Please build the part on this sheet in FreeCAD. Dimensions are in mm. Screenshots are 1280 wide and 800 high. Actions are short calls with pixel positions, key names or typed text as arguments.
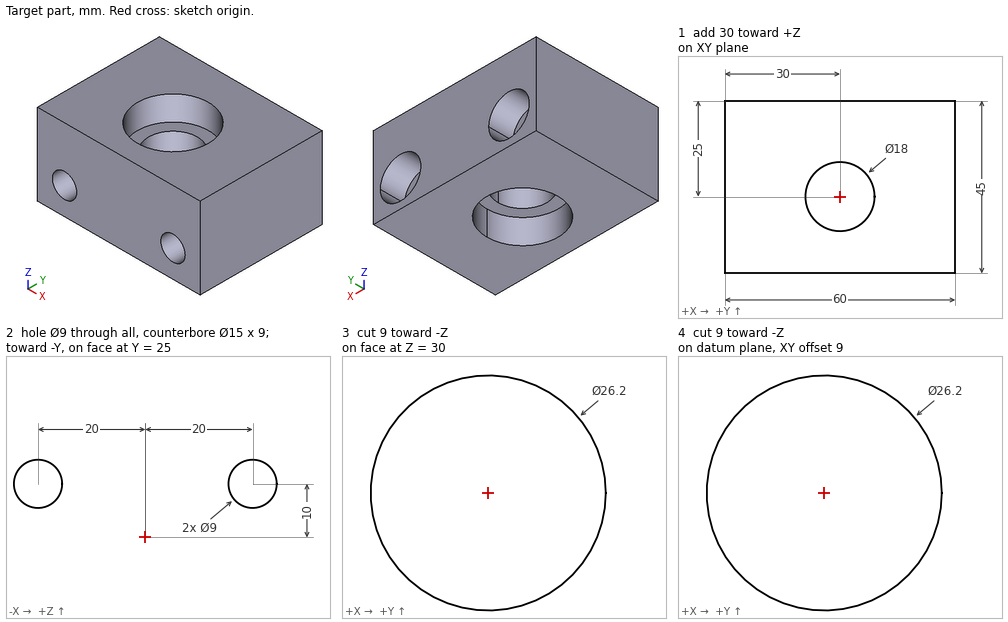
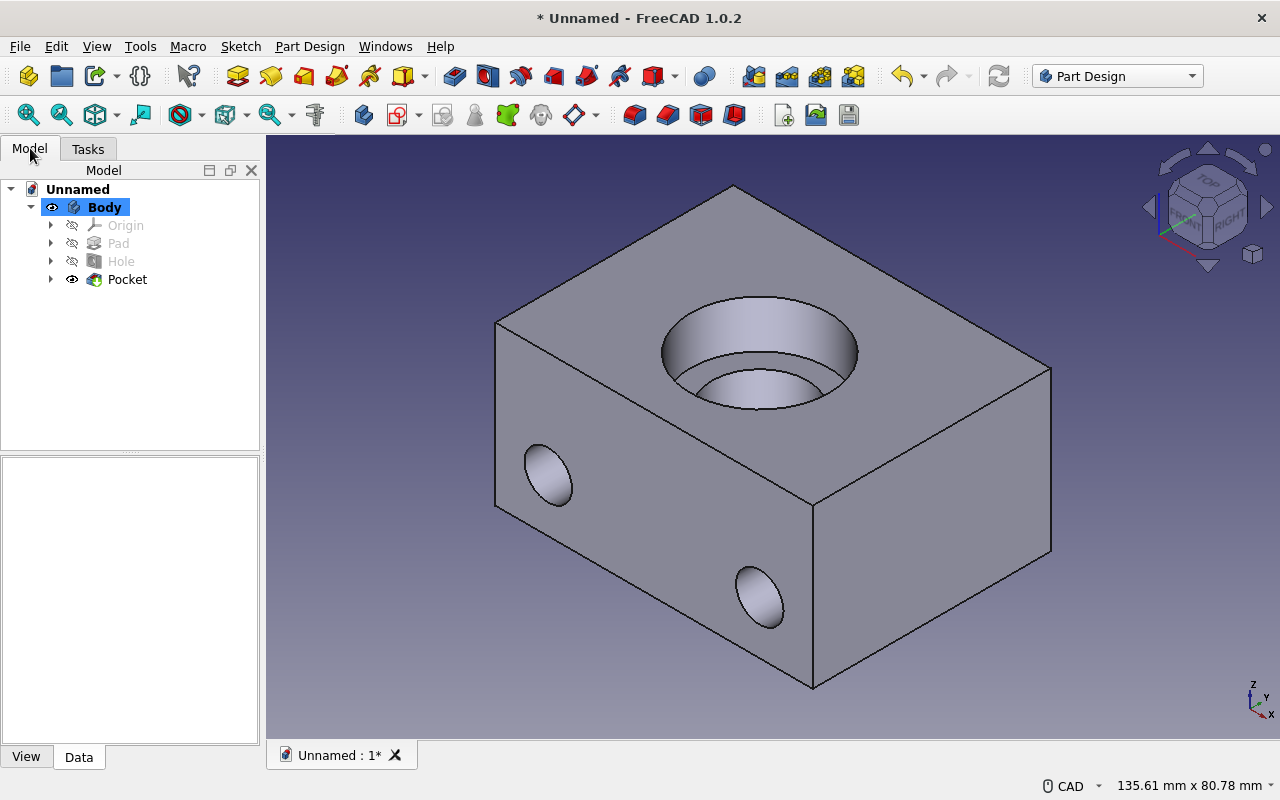
click(51, 225)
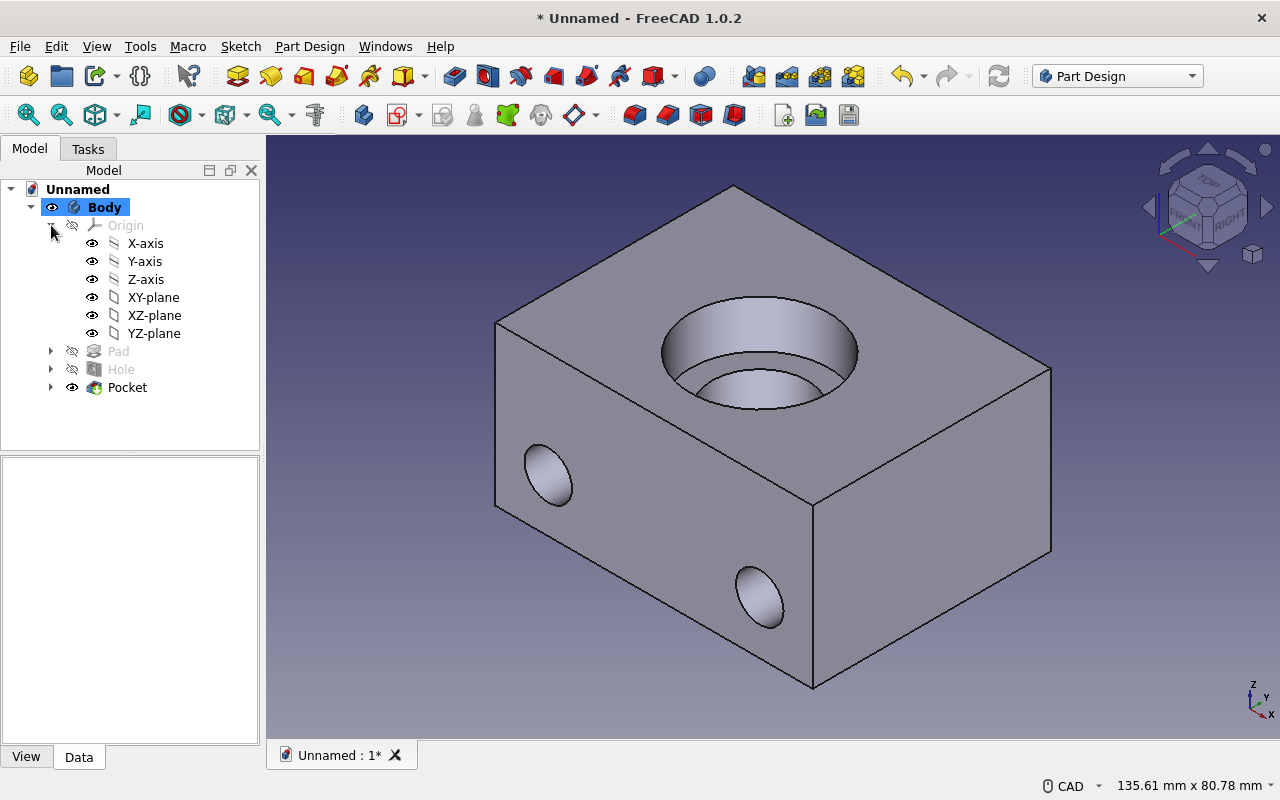
click(137, 297)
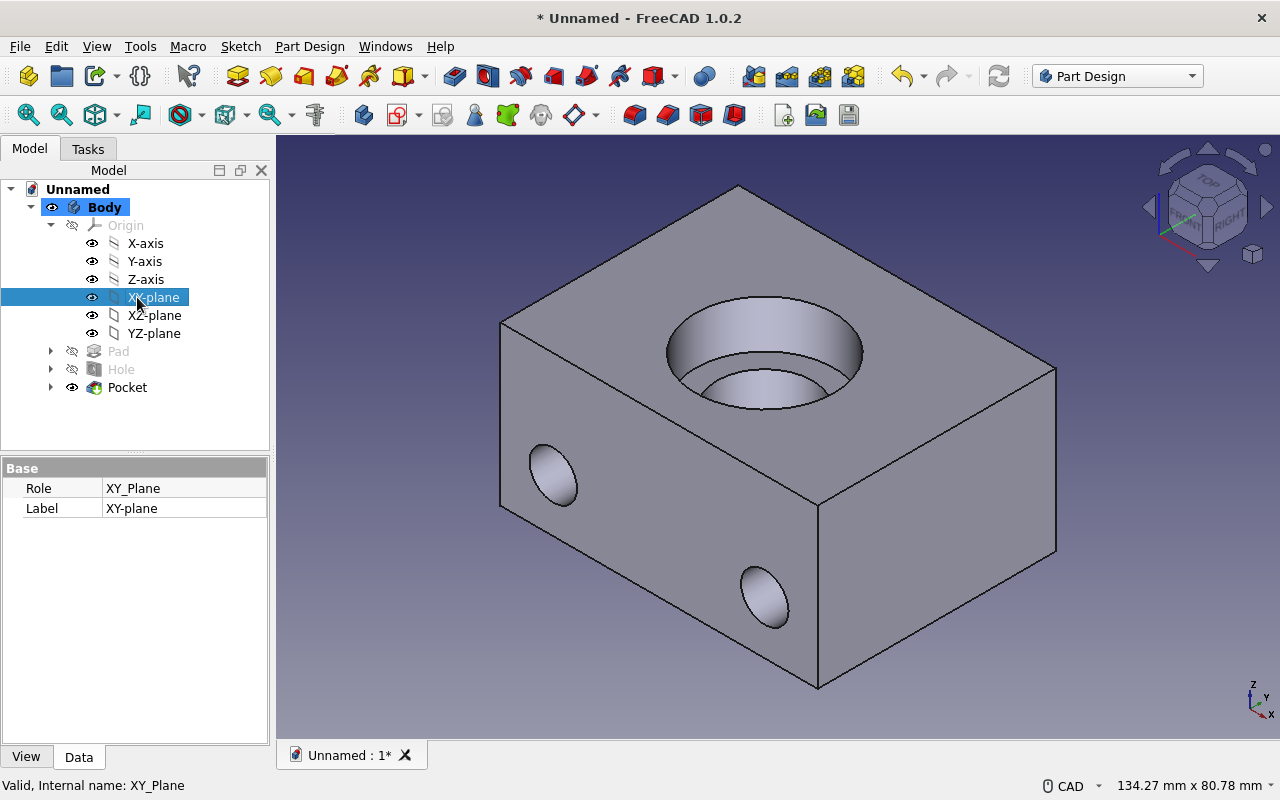
click(574, 116)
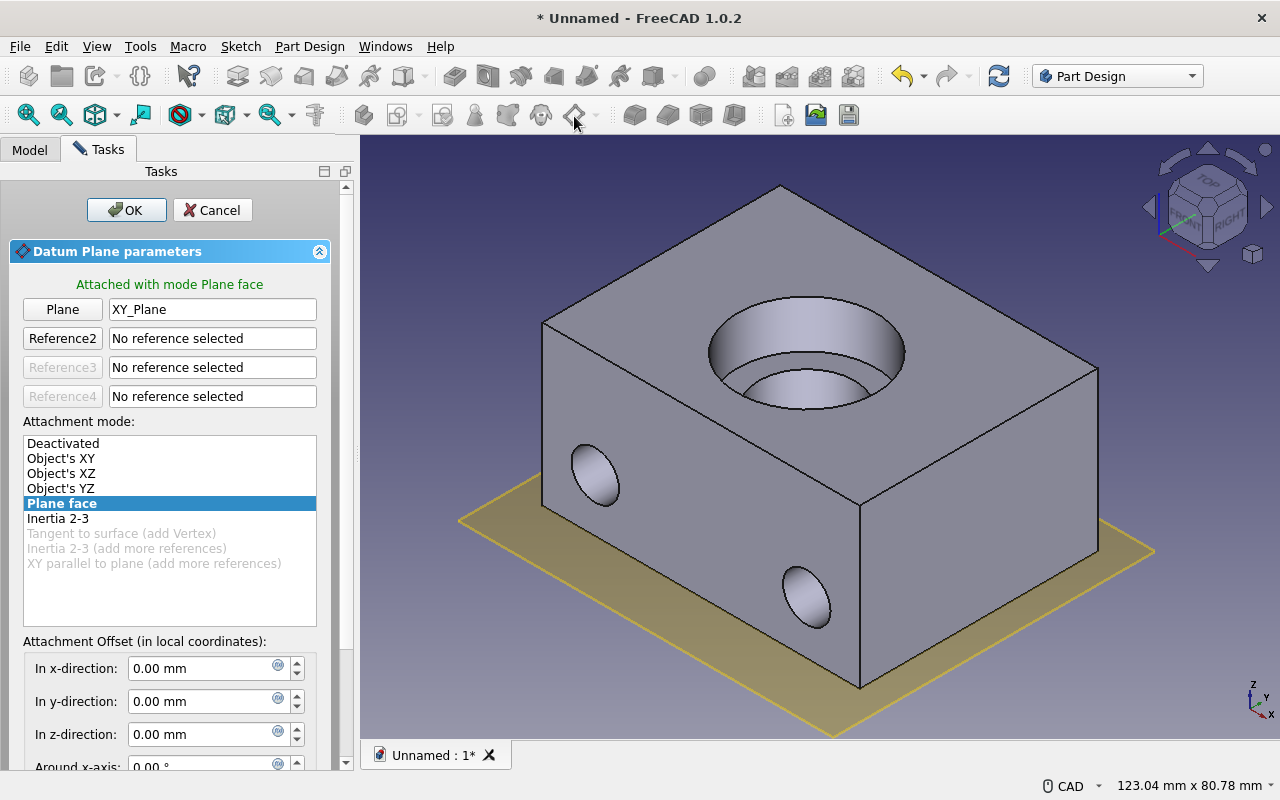
triple_click(210, 734)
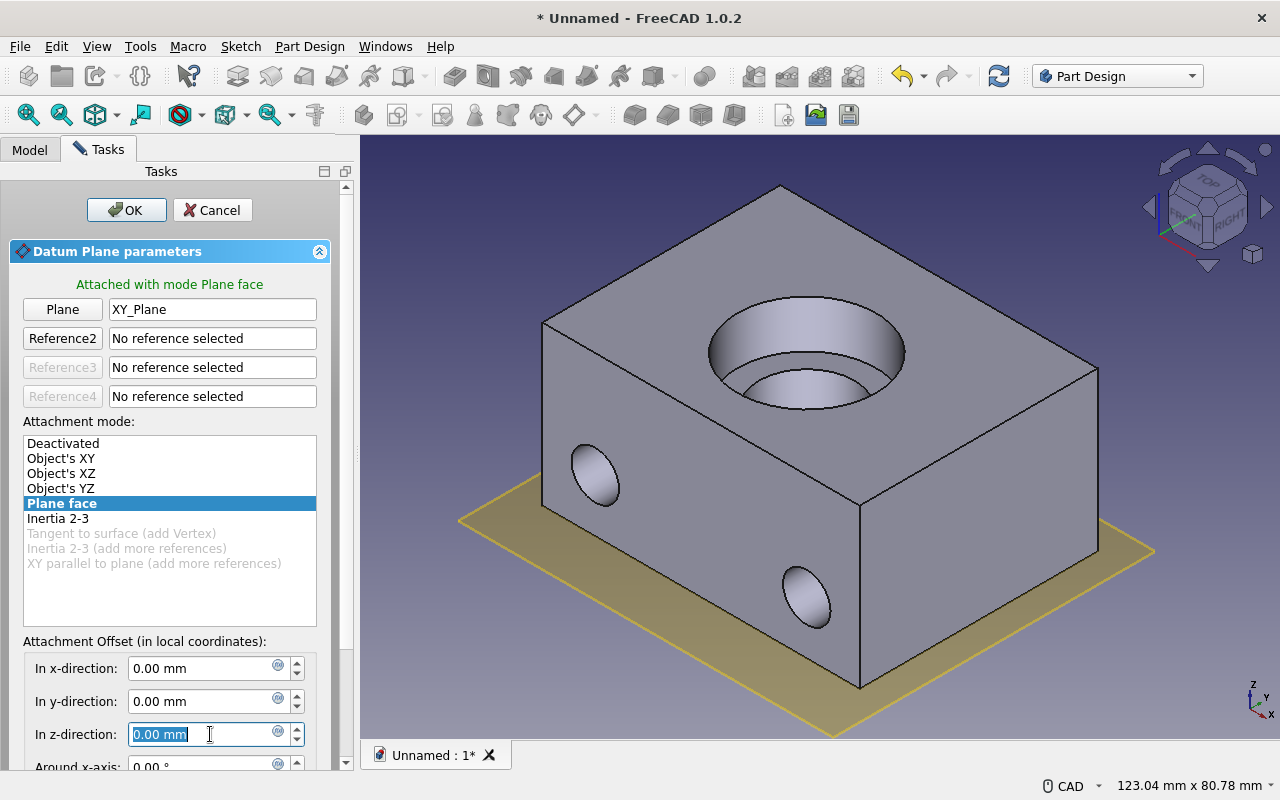
text(9)
key(Tab)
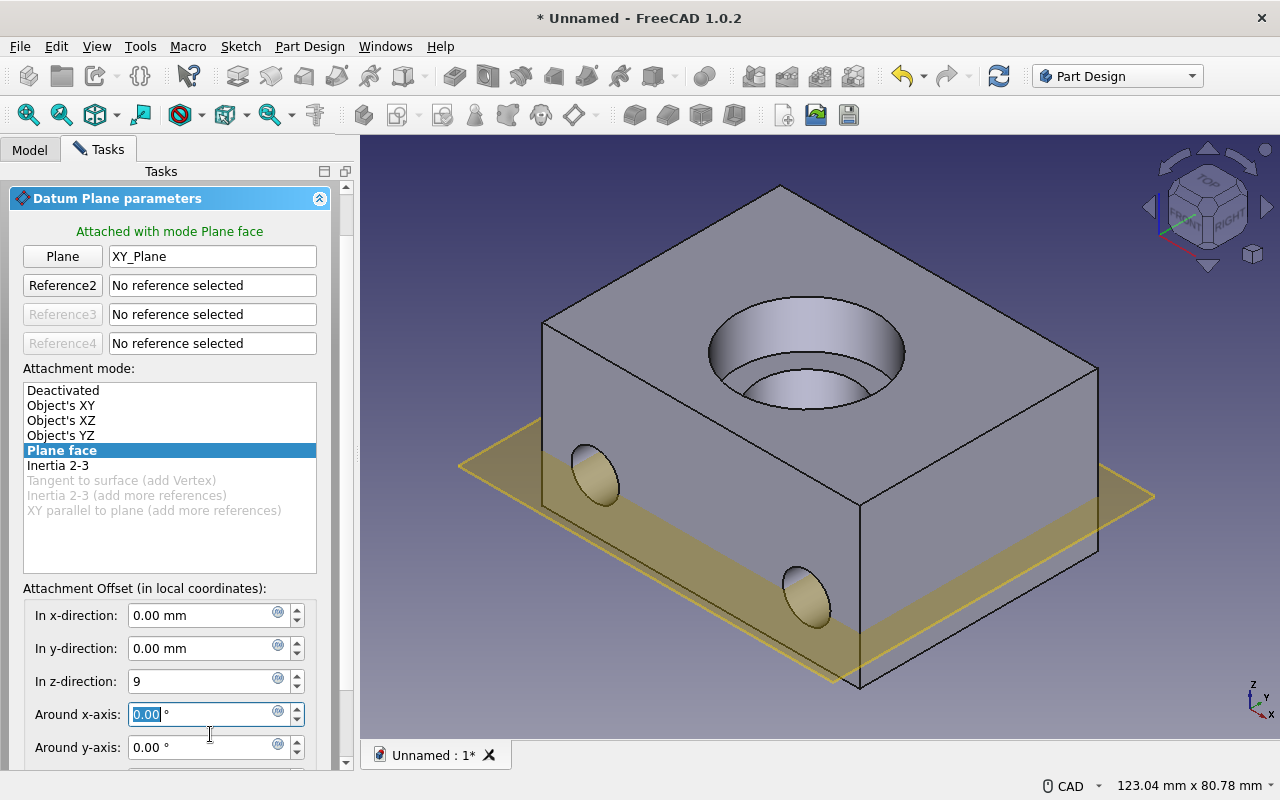
scroll(346, 476, up, 2)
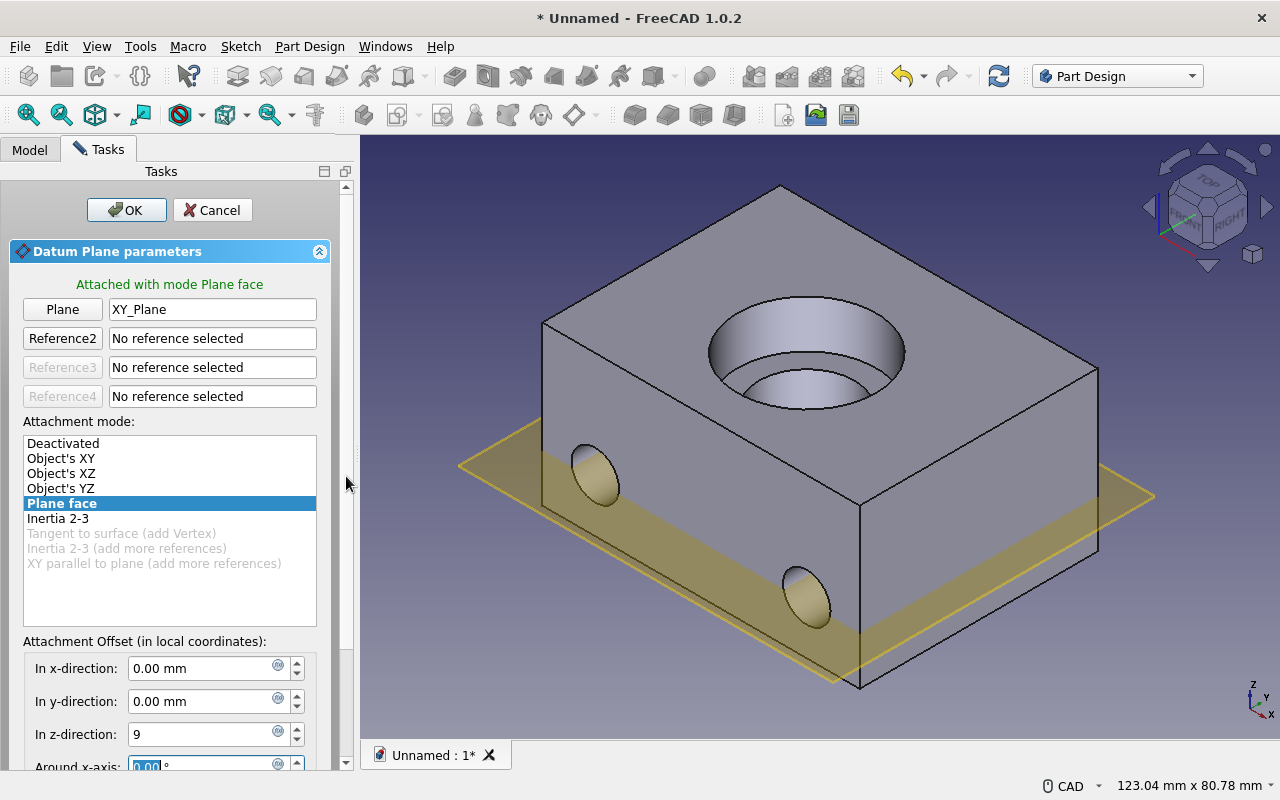
click(127, 210)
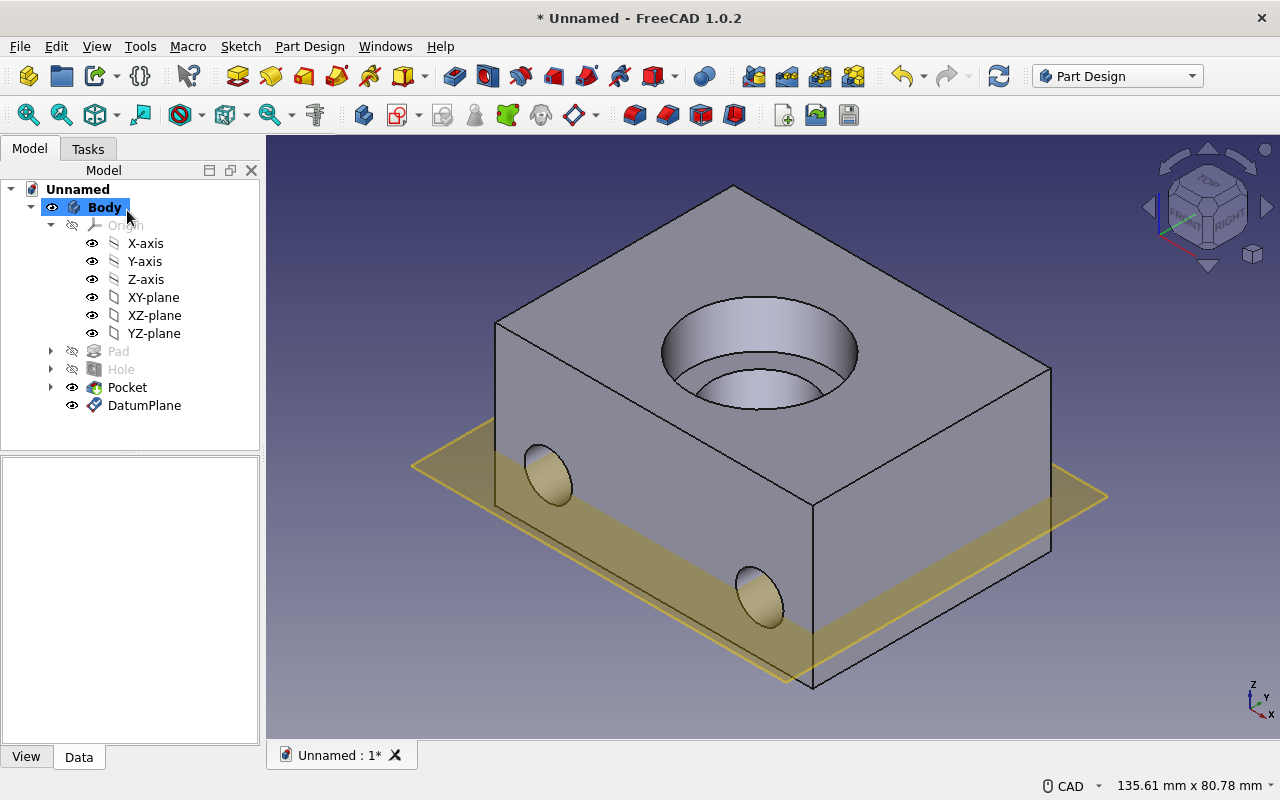
click(117, 405)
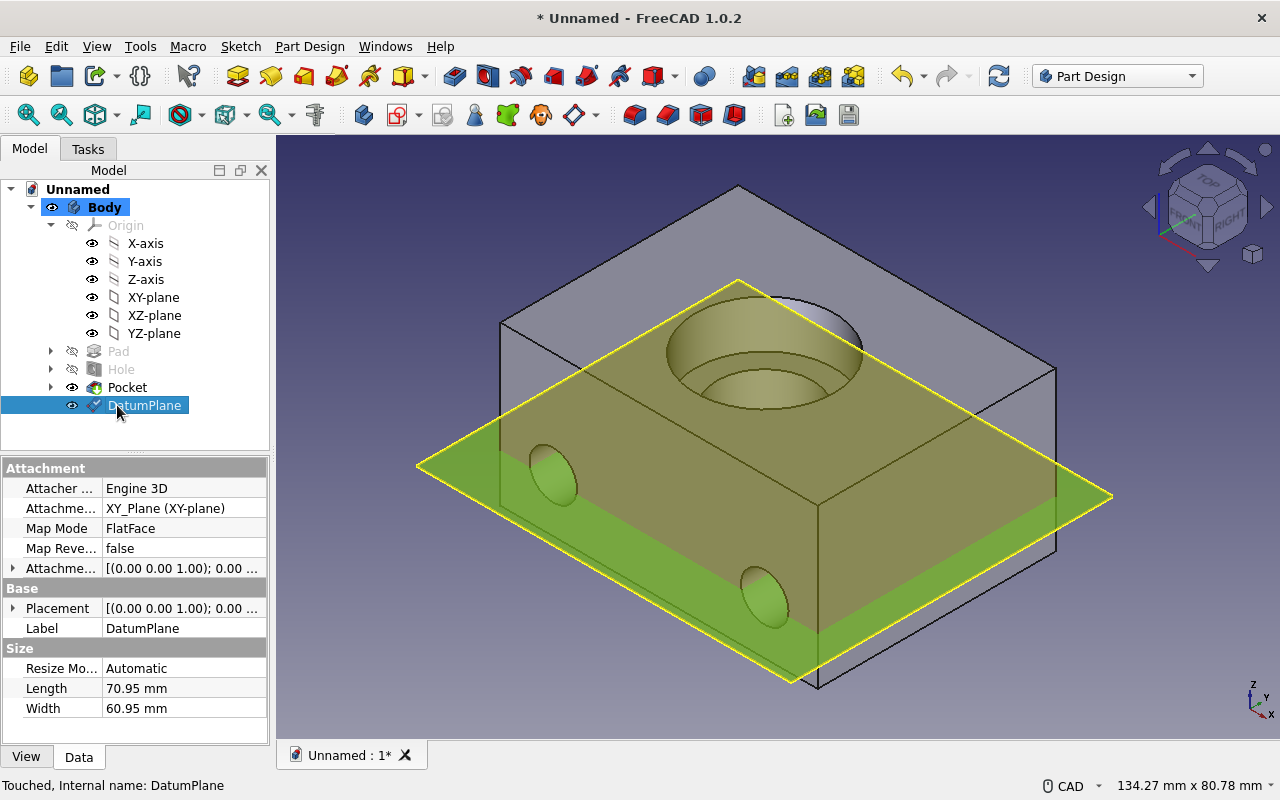
click(396, 116)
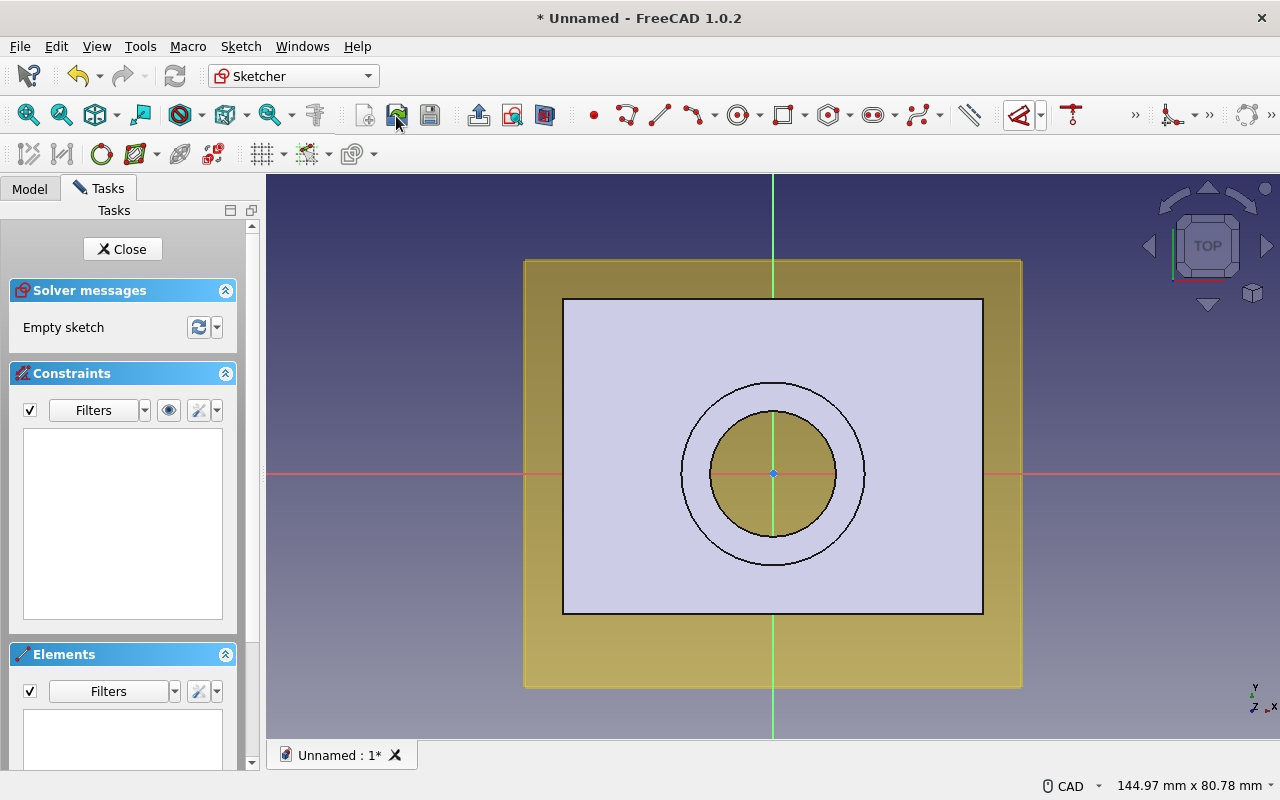
click(545, 116)